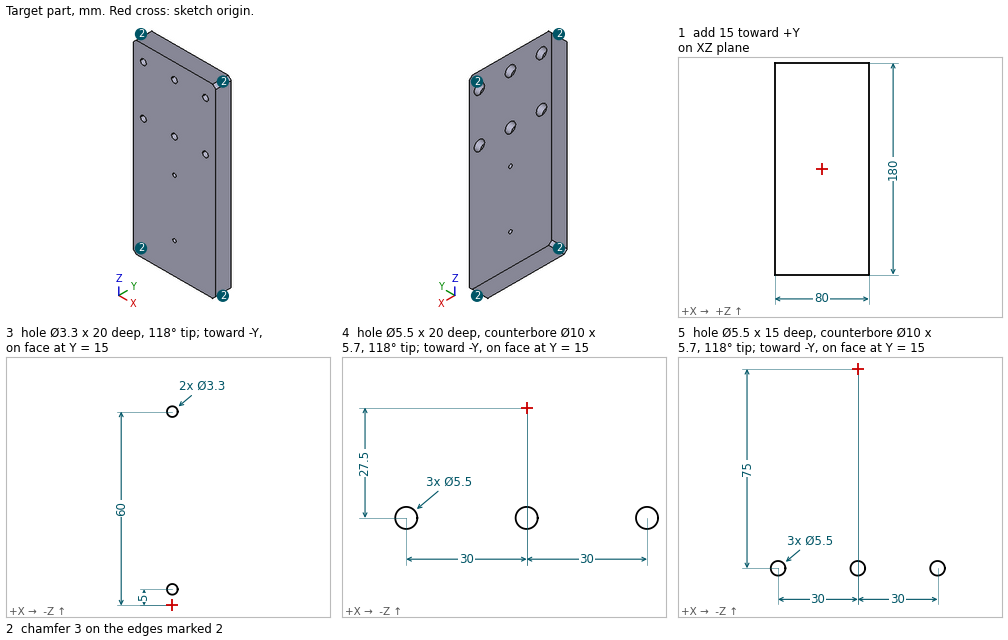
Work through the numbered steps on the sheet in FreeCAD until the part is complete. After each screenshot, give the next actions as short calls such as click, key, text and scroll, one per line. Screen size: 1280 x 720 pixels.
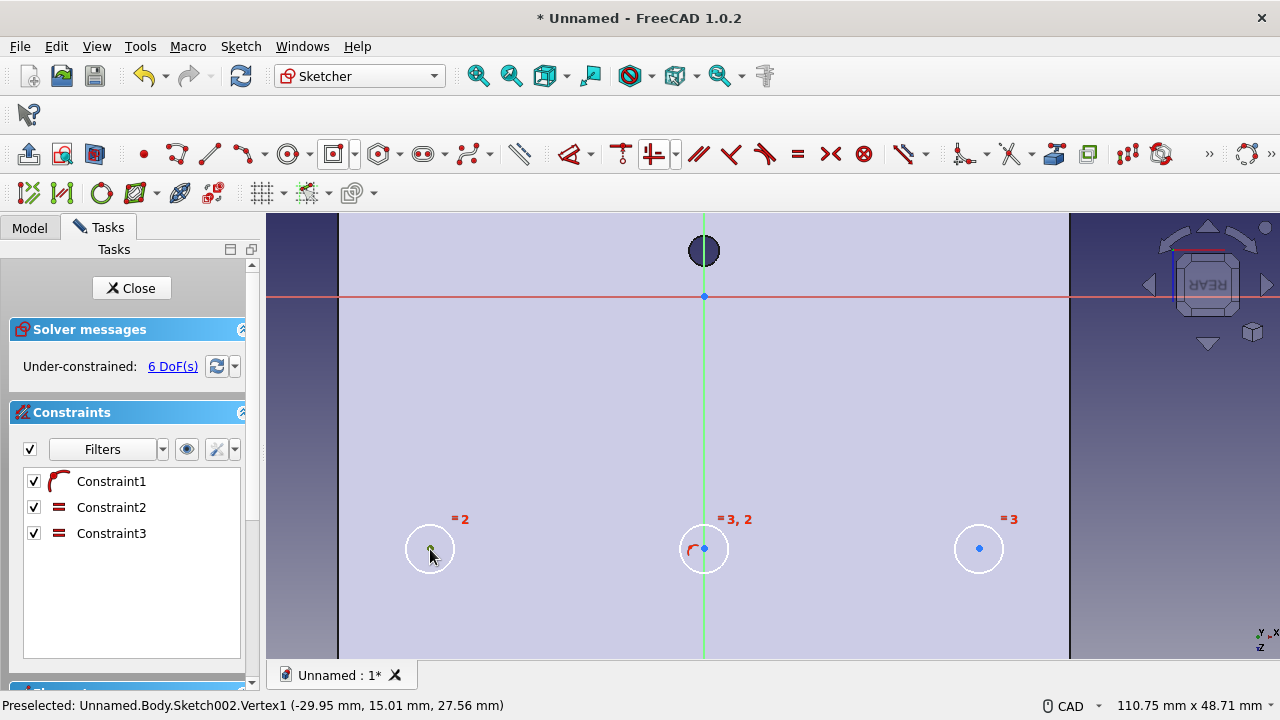
click(704, 549)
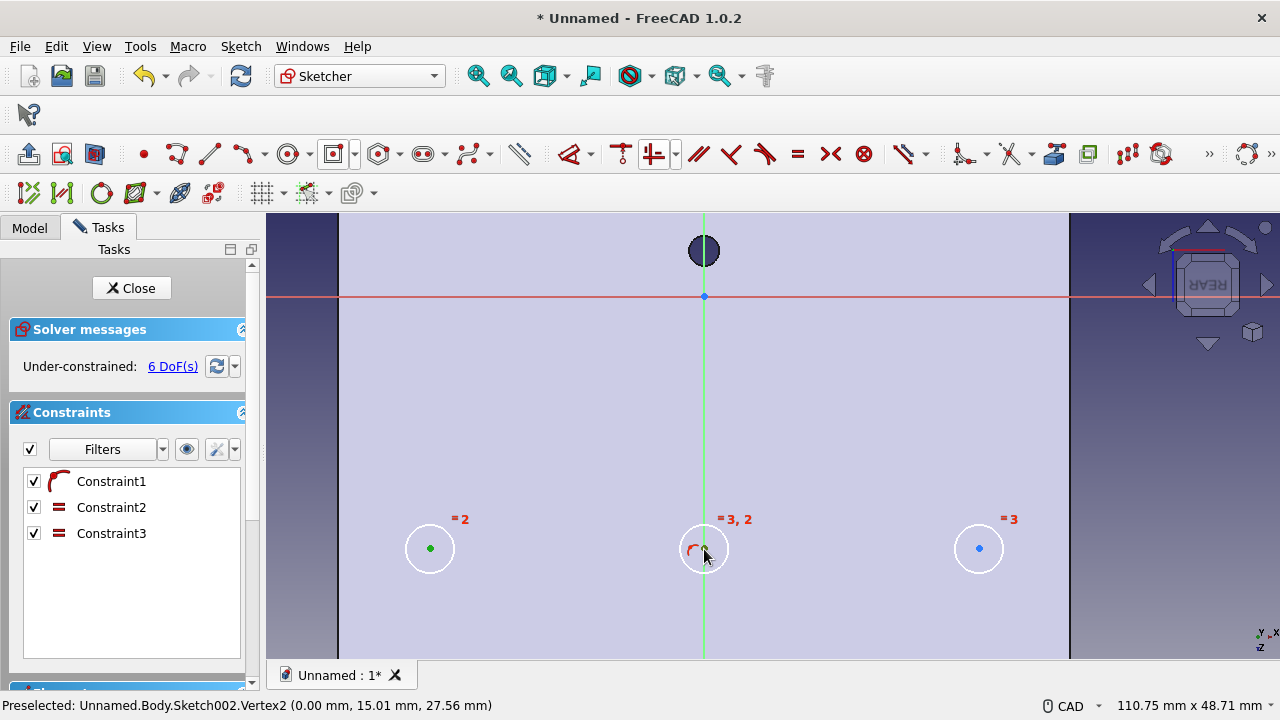
key(h)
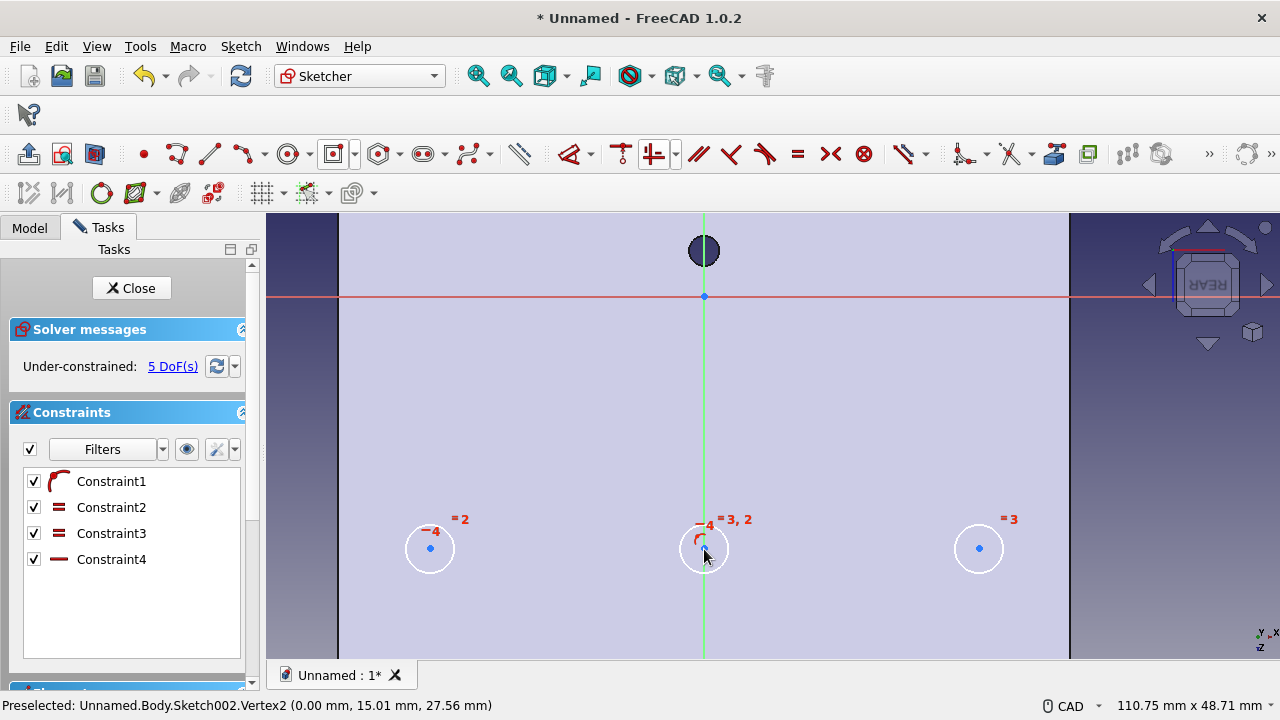
click(704, 549)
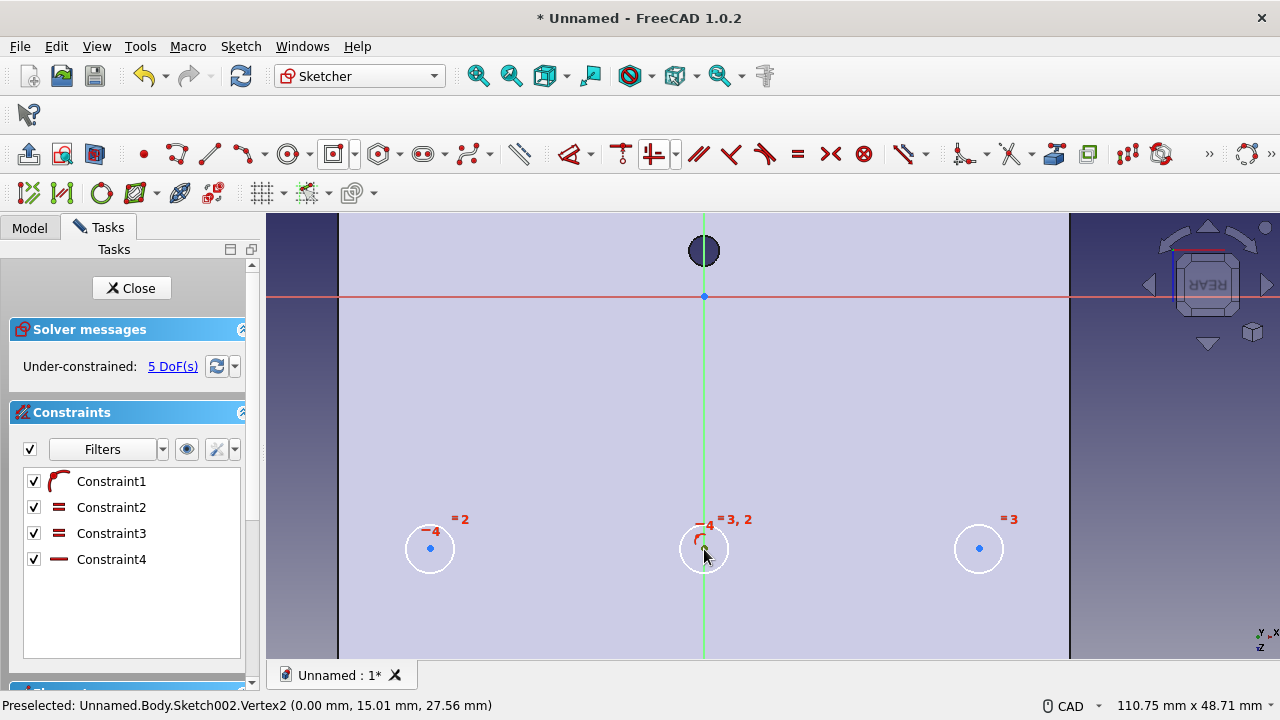
click(979, 549)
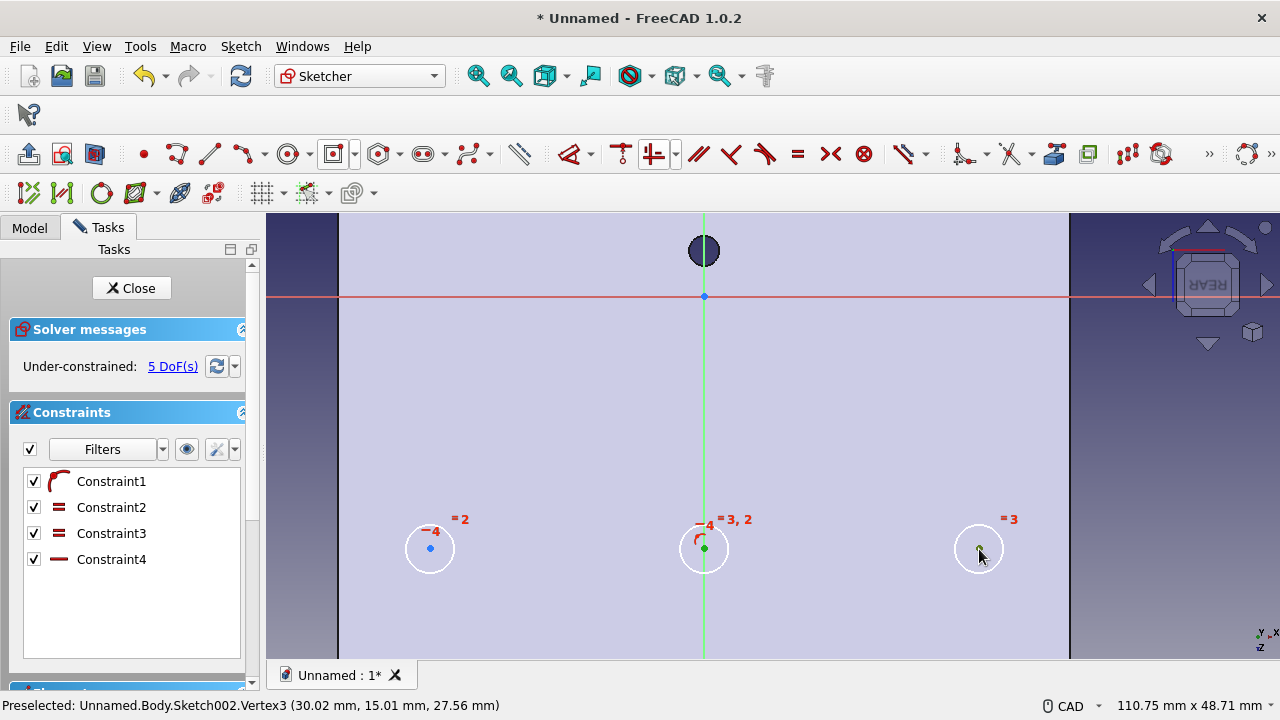
key(h)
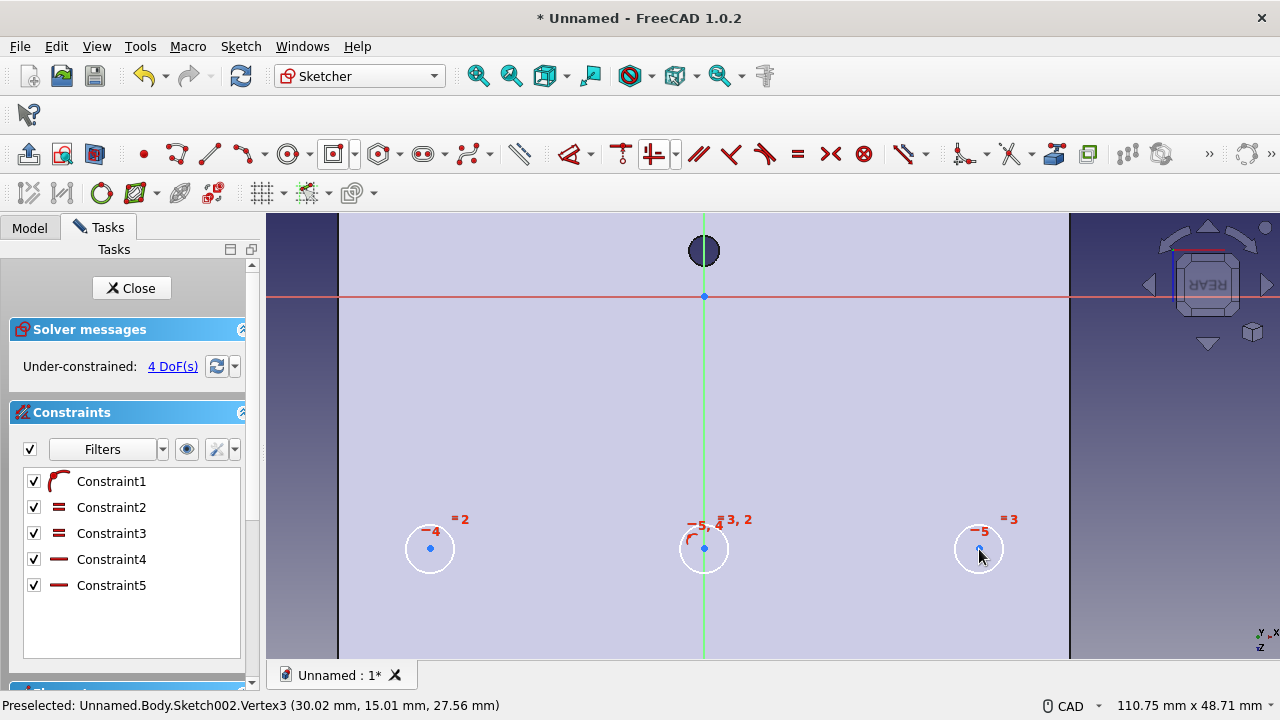
click(568, 154)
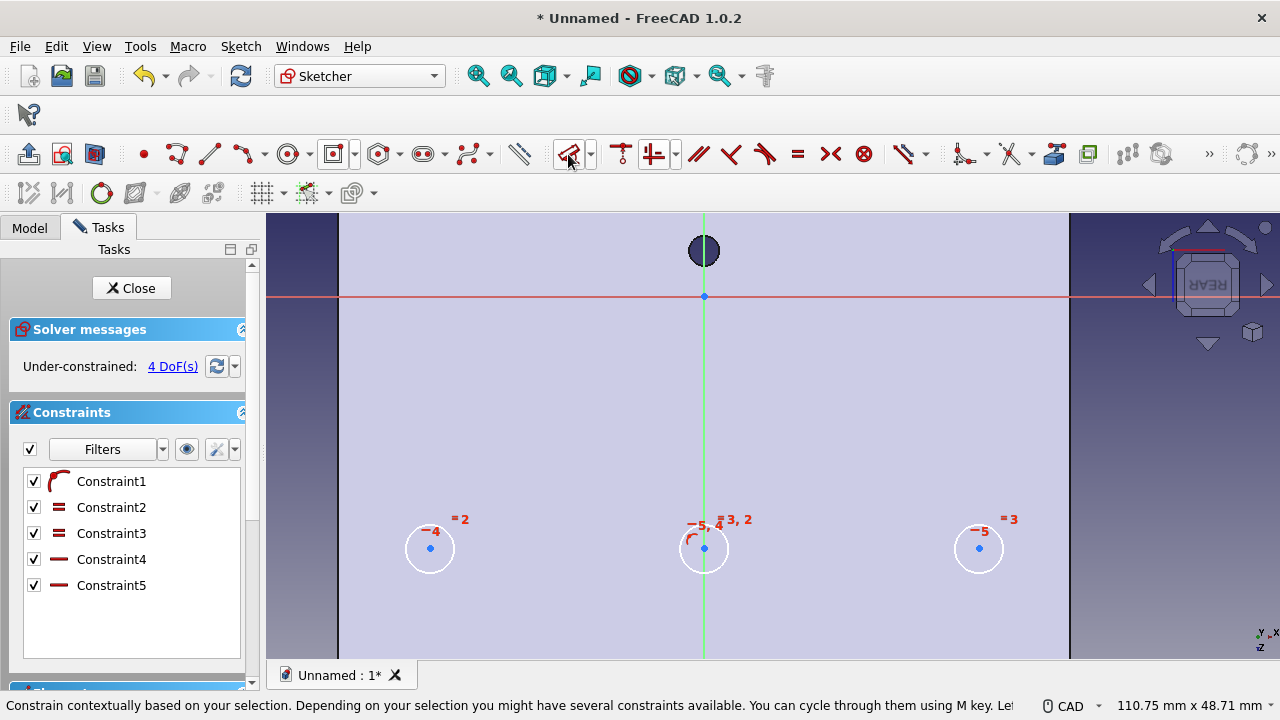
click(447, 532)
click(470, 509)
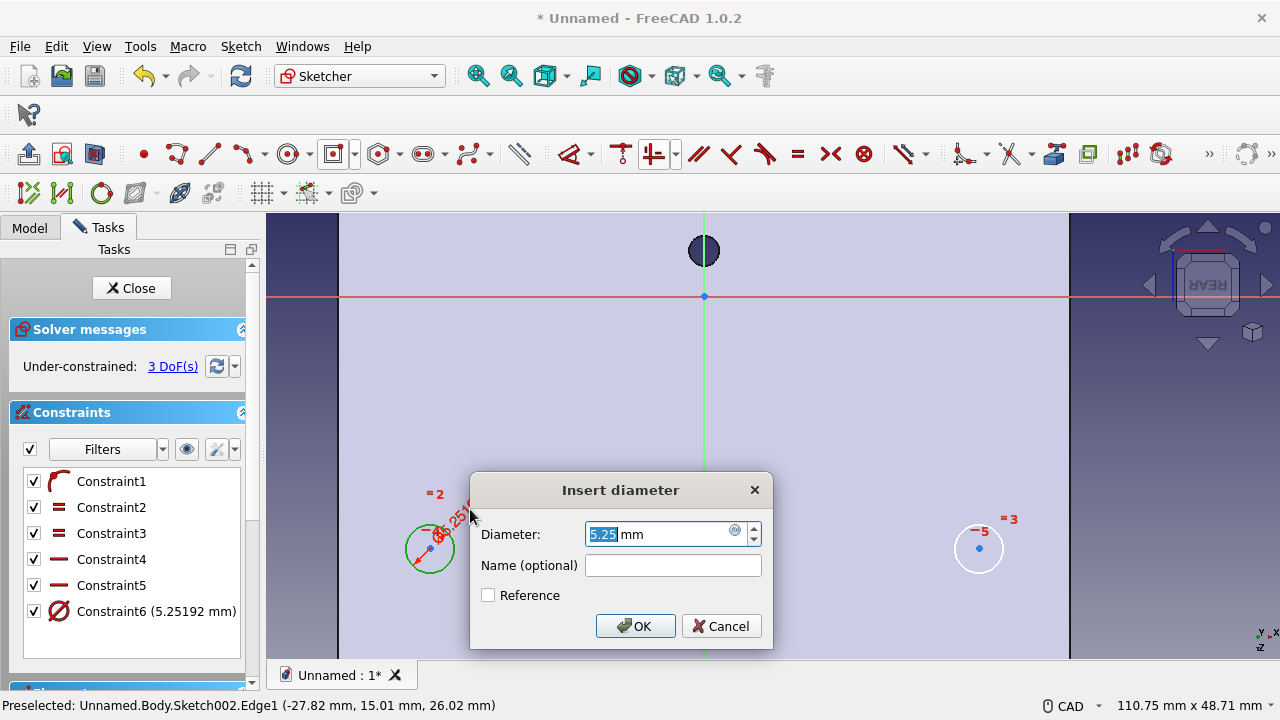
text(5.5)
key(Return)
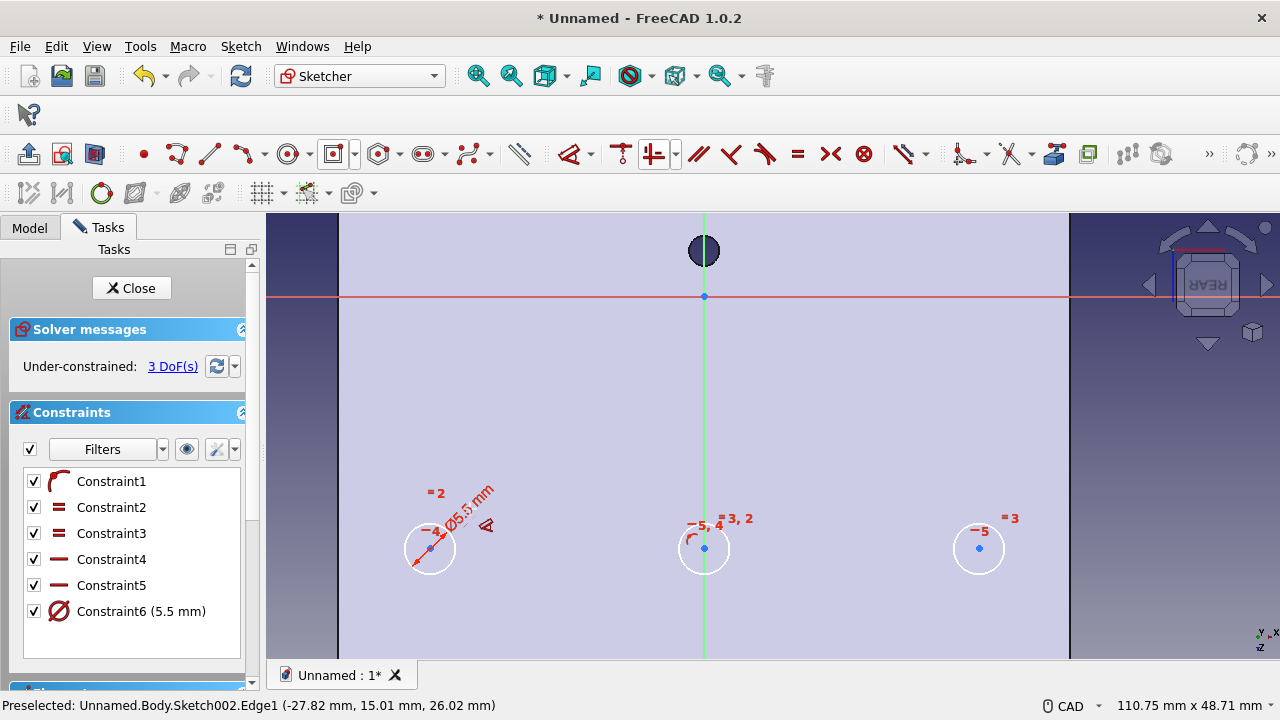
click(430, 549)
click(567, 263)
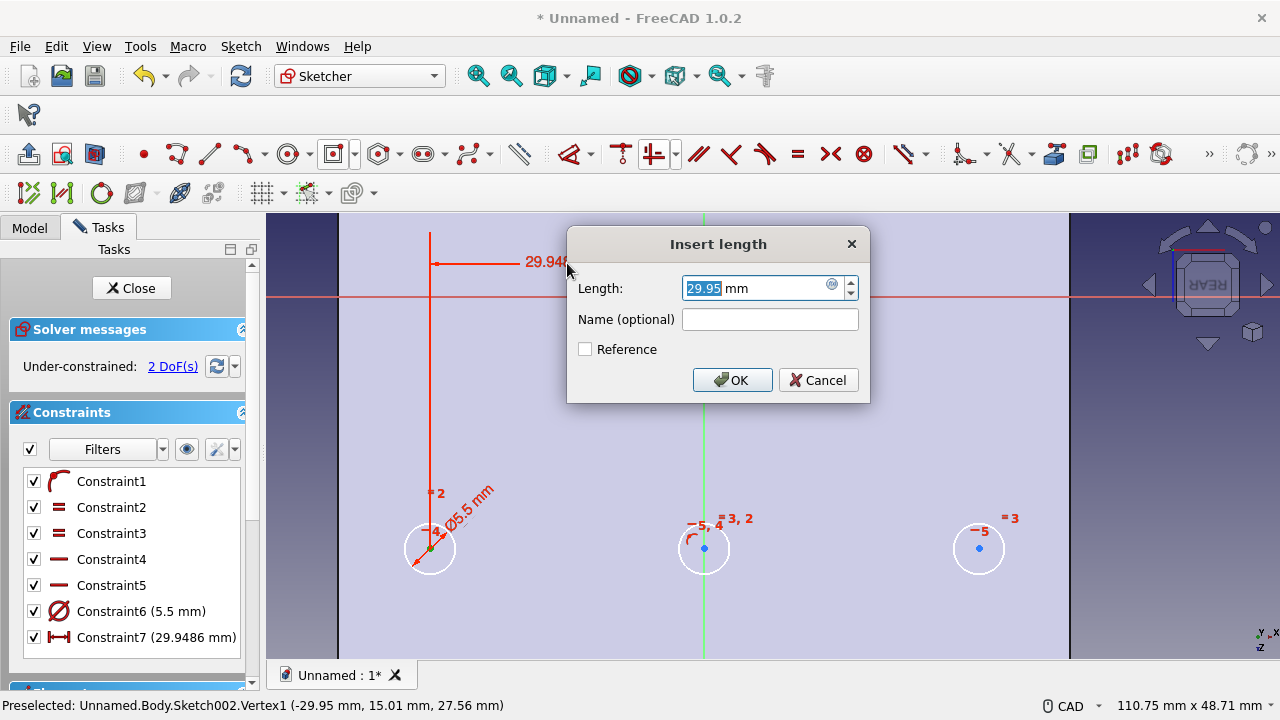
text(30)
key(Return)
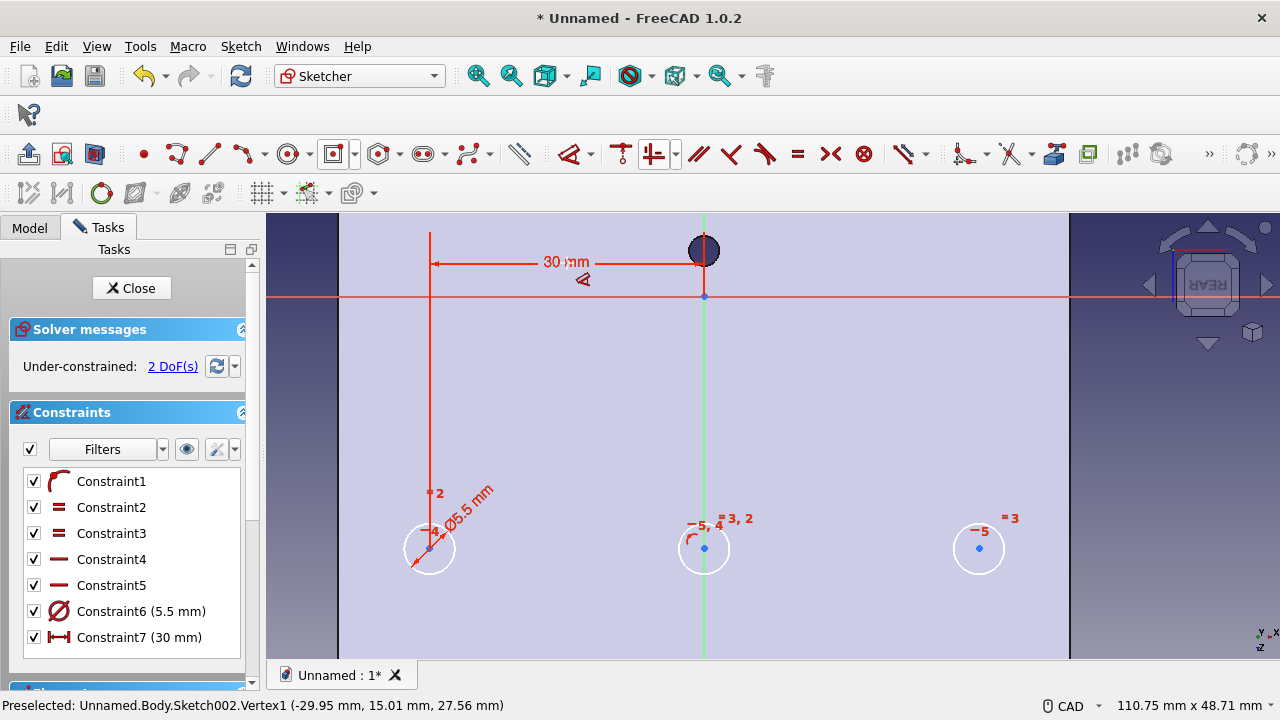
click(979, 549)
click(842, 263)